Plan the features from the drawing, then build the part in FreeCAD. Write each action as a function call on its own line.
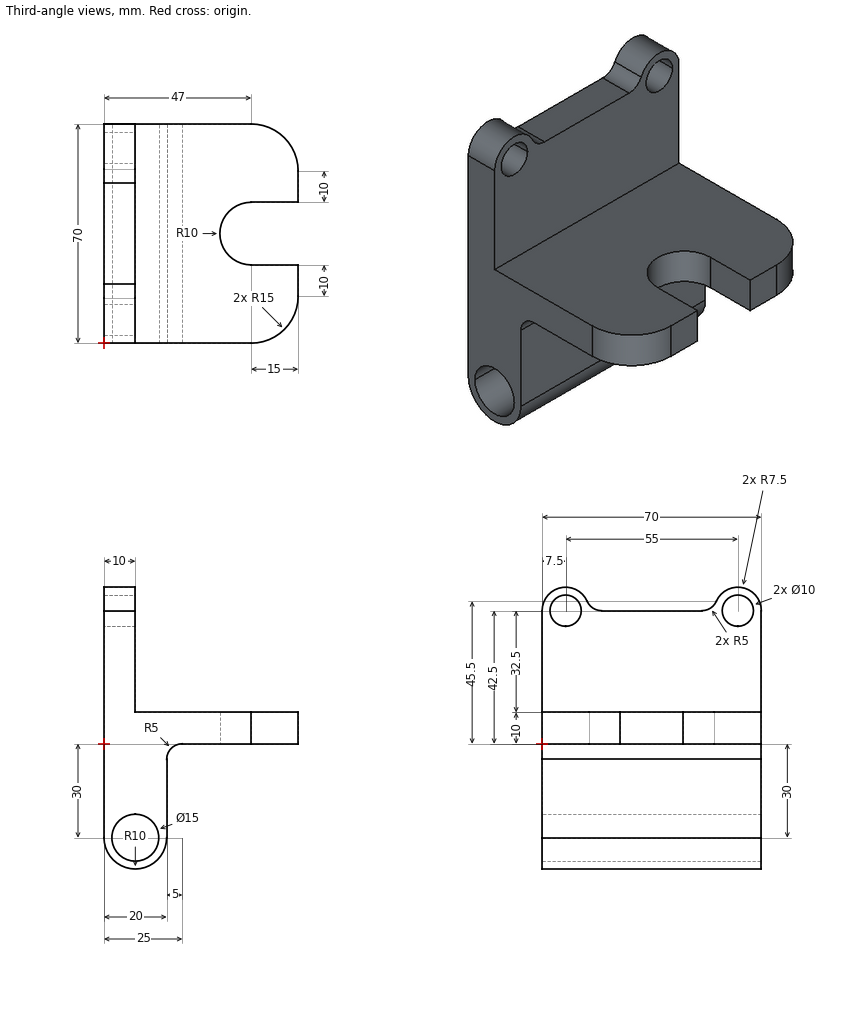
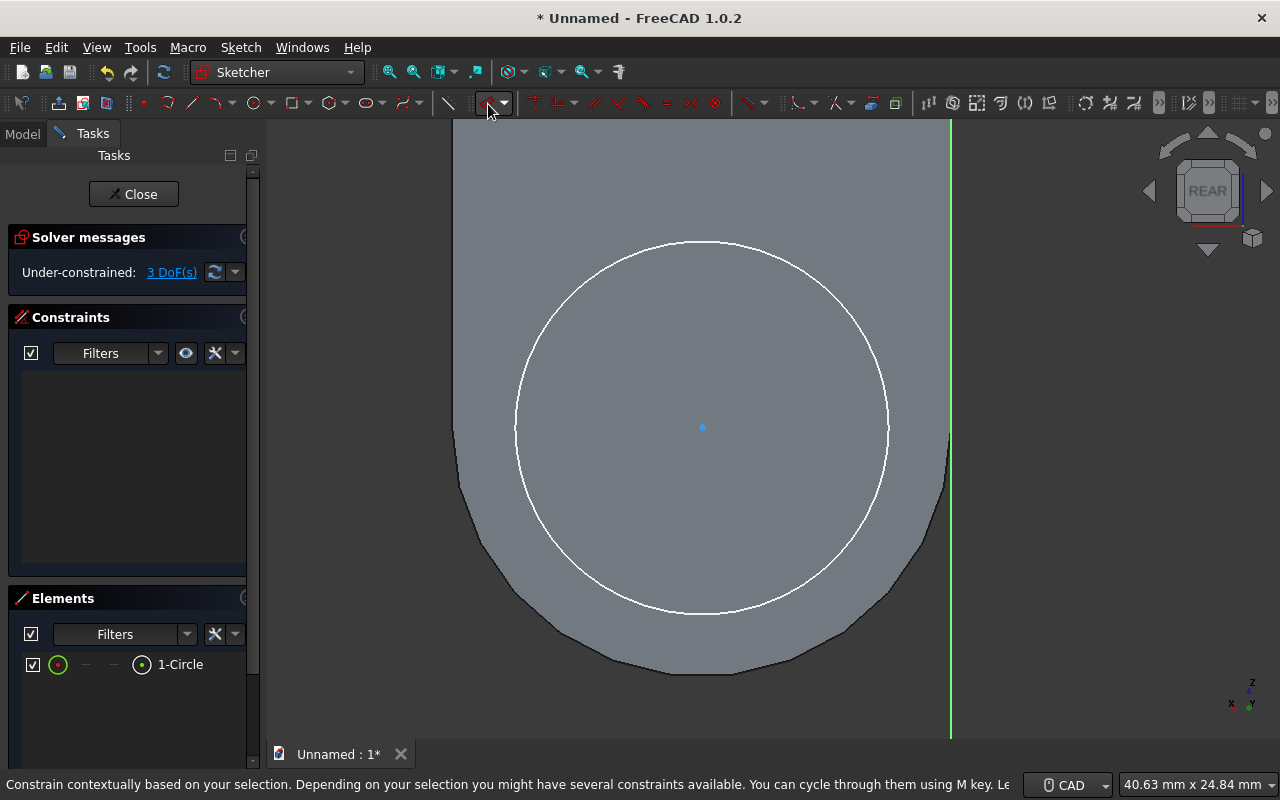
click(834, 296)
click(857, 273)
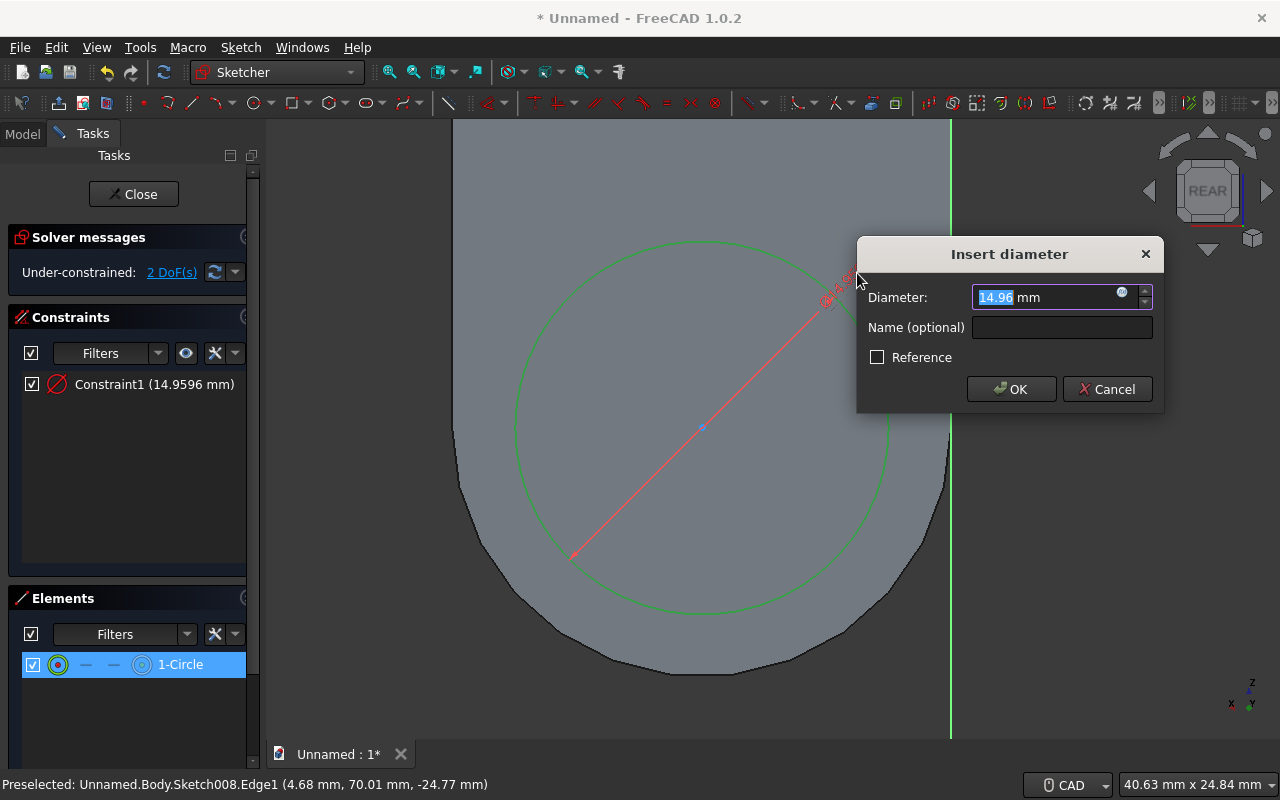
text(15)
key(Return)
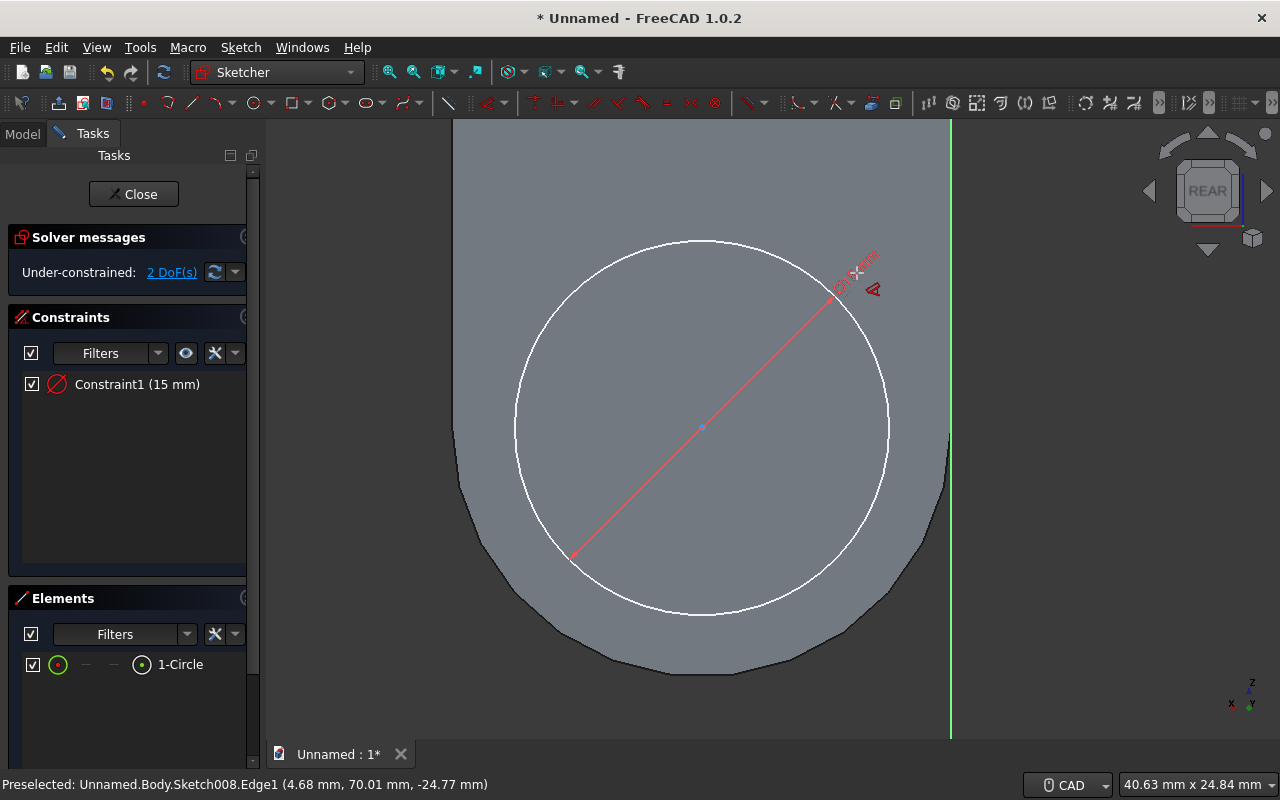
click(702, 428)
click(827, 462)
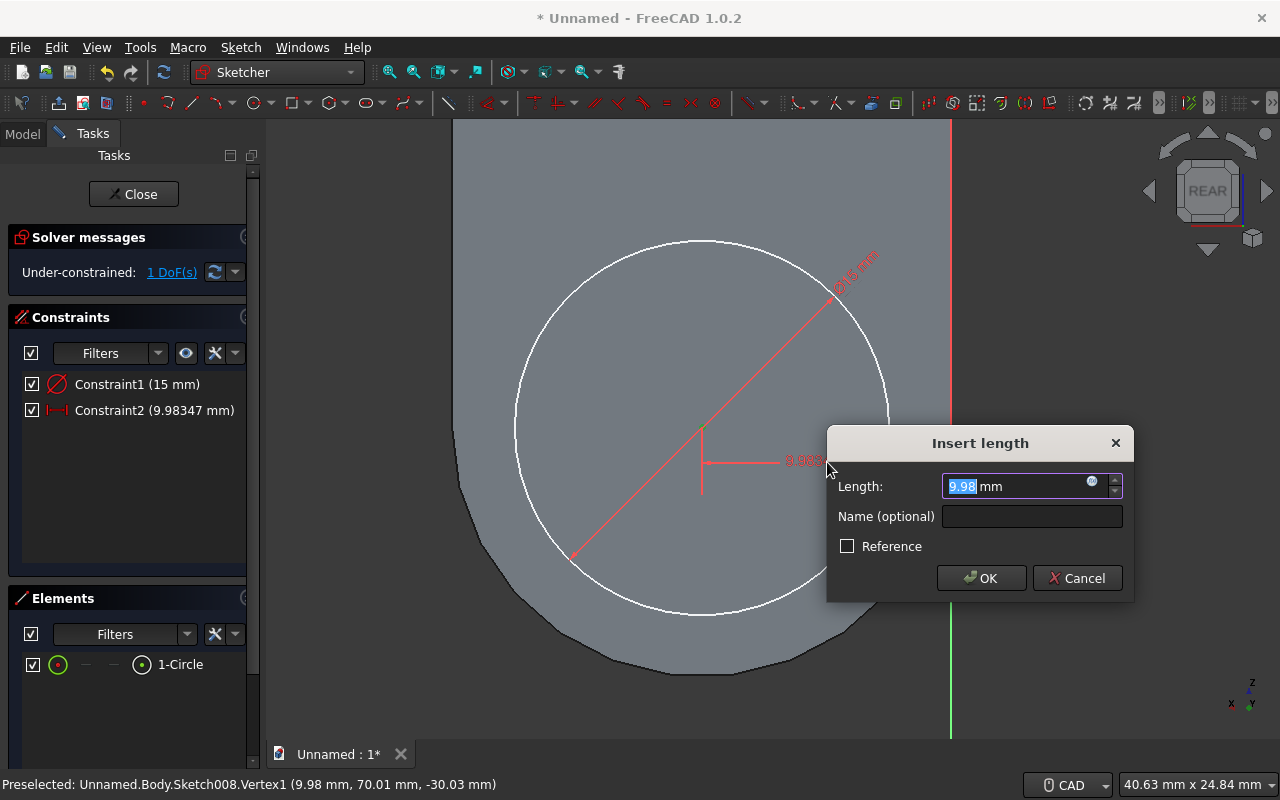
text(10)
key(Return)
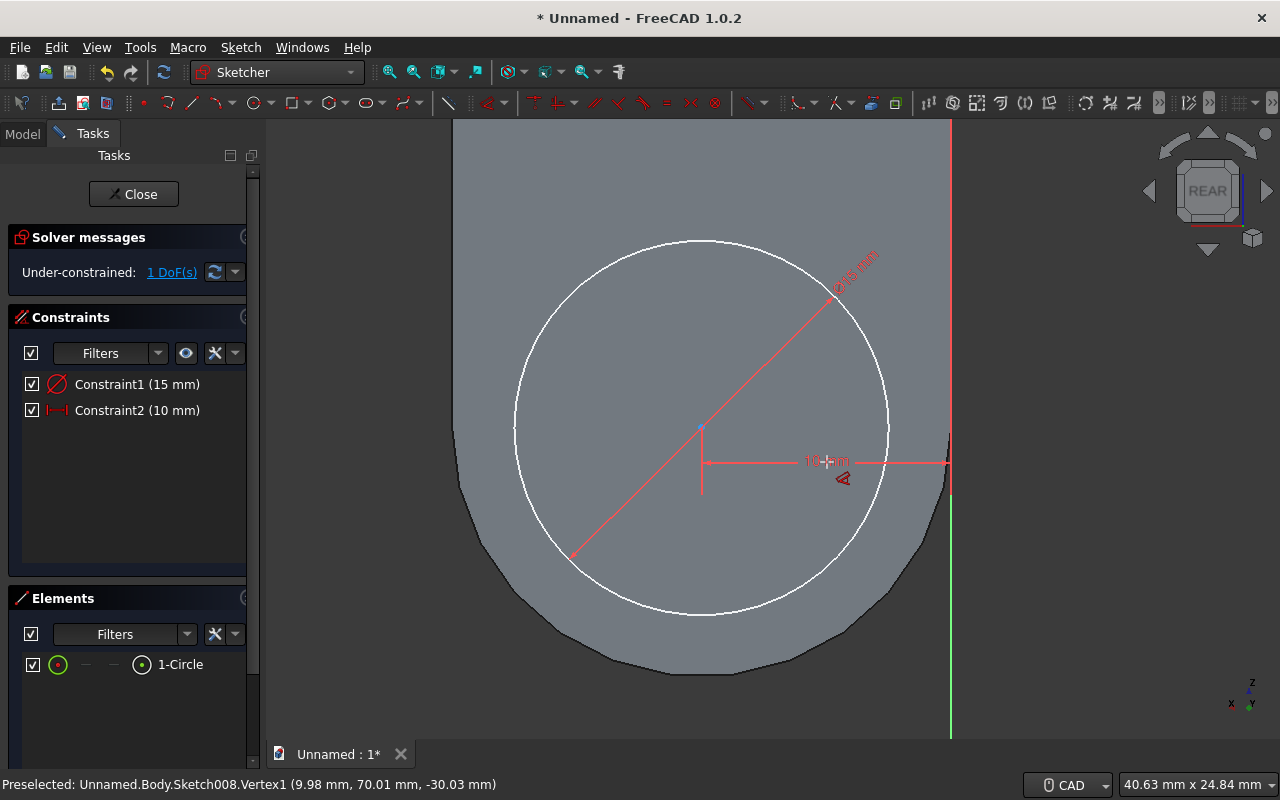
click(702, 428)
click(985, 288)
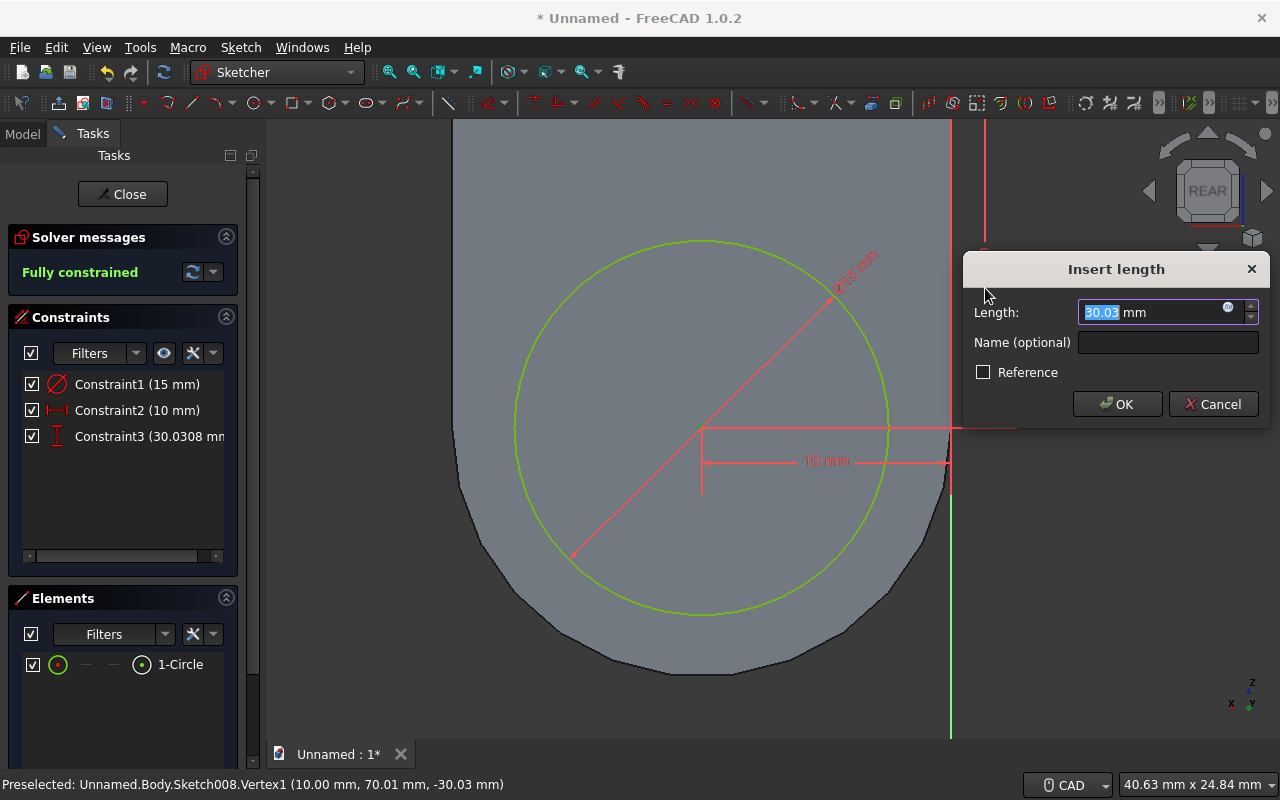
text(30)
key(Return)
key(Escape)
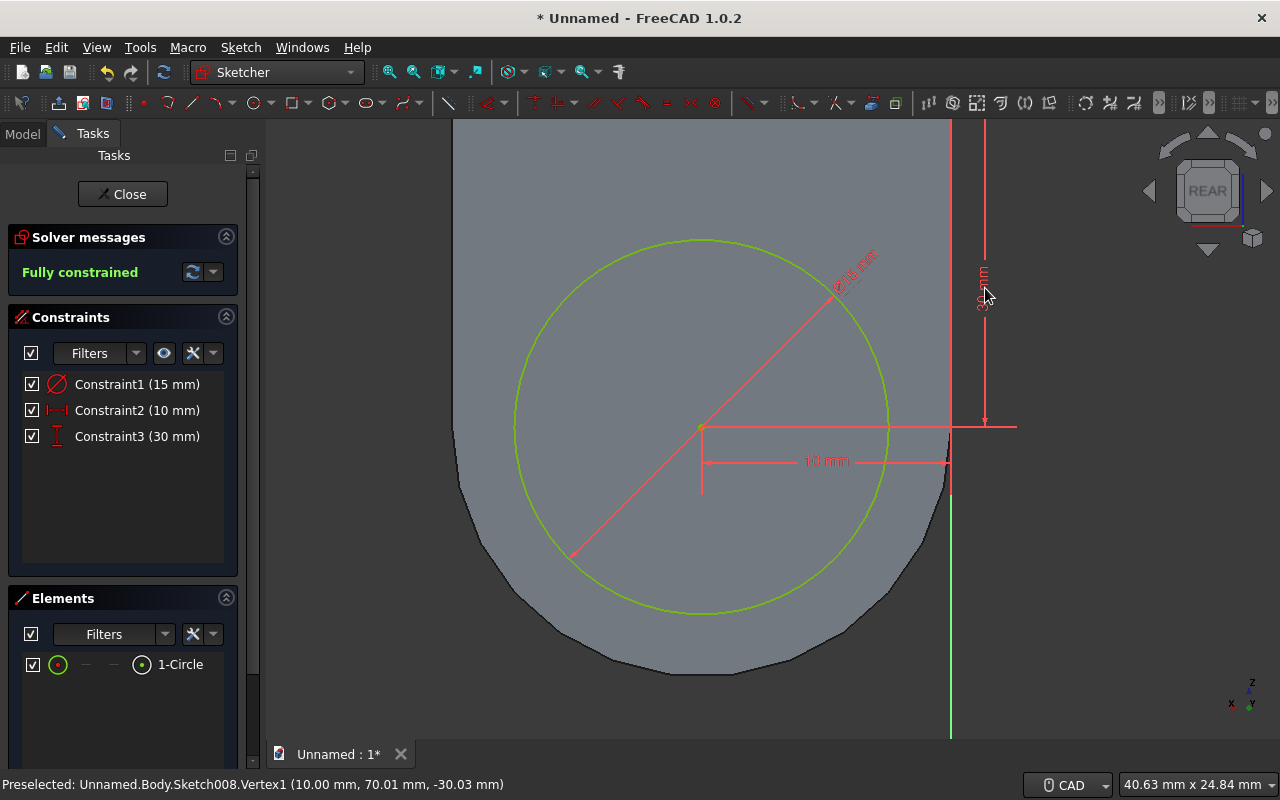
click(123, 194)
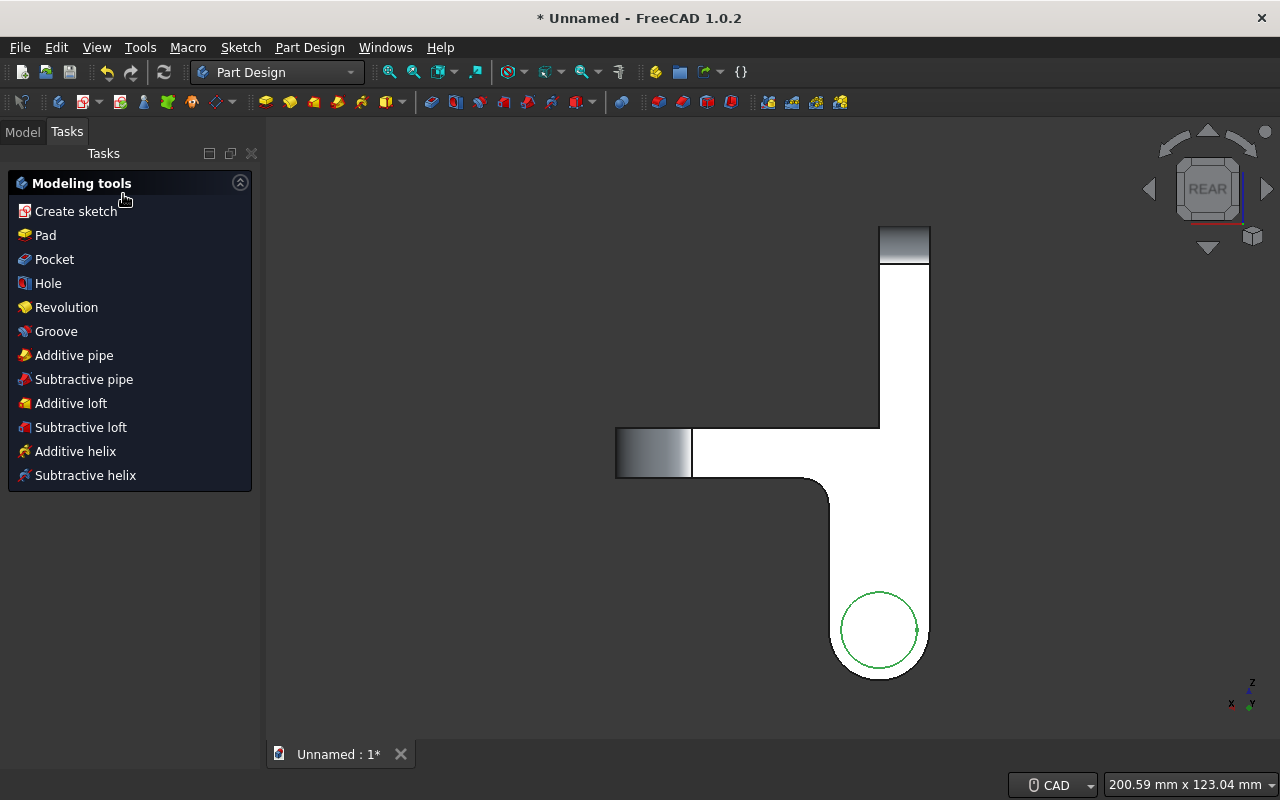
click(432, 102)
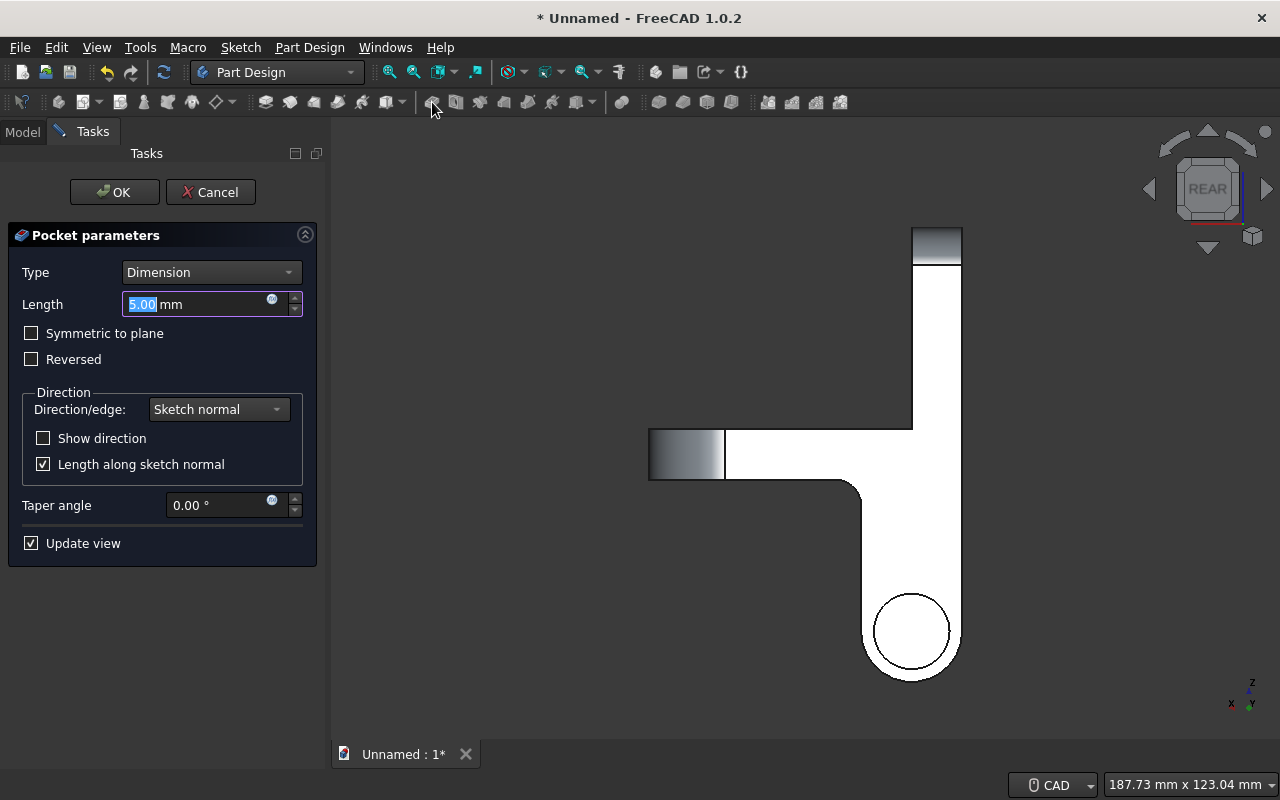
text(70)
key(Tab)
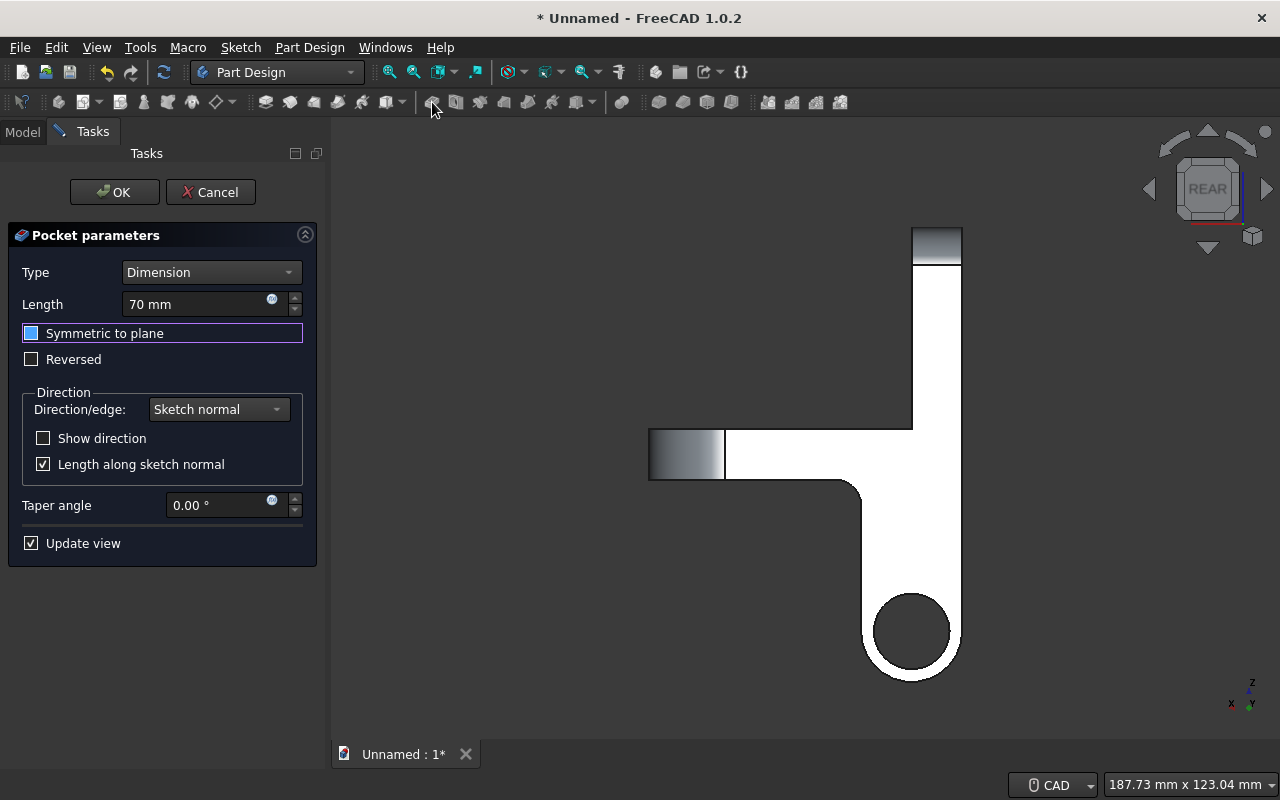
click(115, 192)